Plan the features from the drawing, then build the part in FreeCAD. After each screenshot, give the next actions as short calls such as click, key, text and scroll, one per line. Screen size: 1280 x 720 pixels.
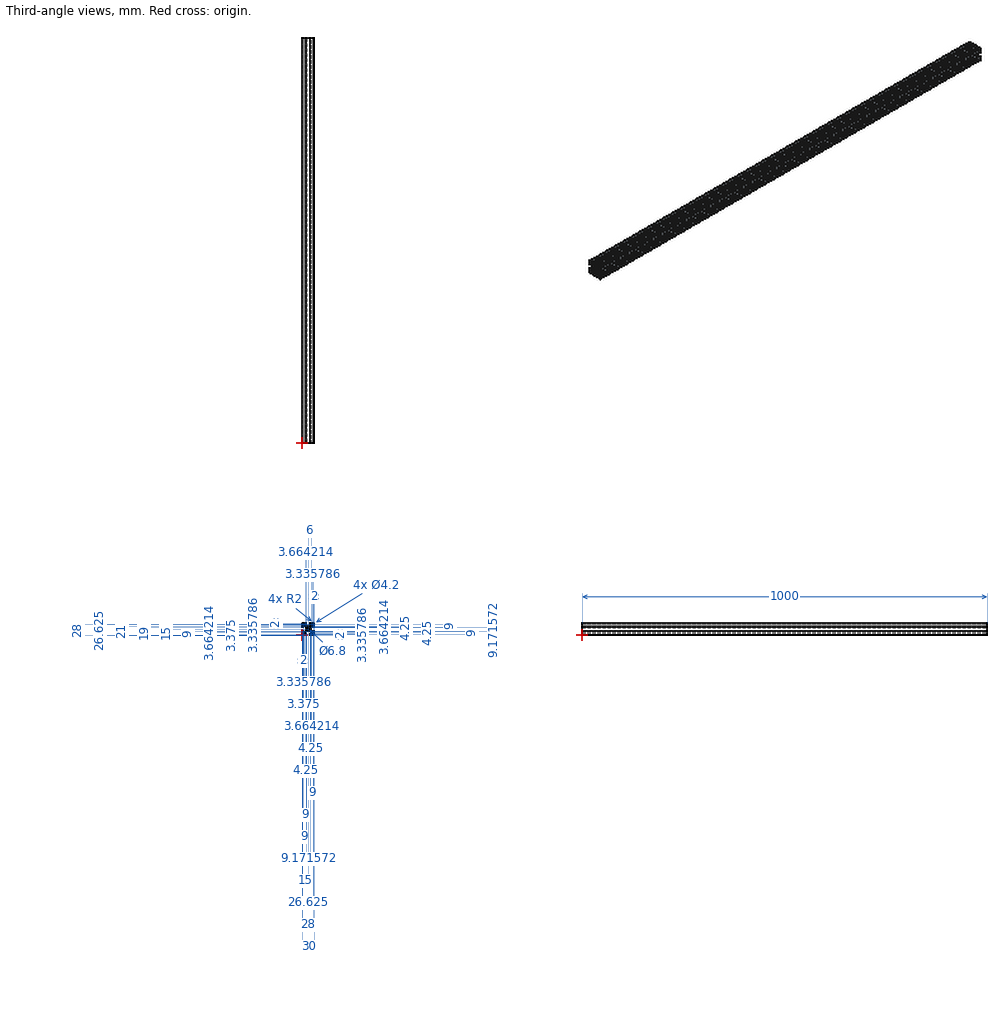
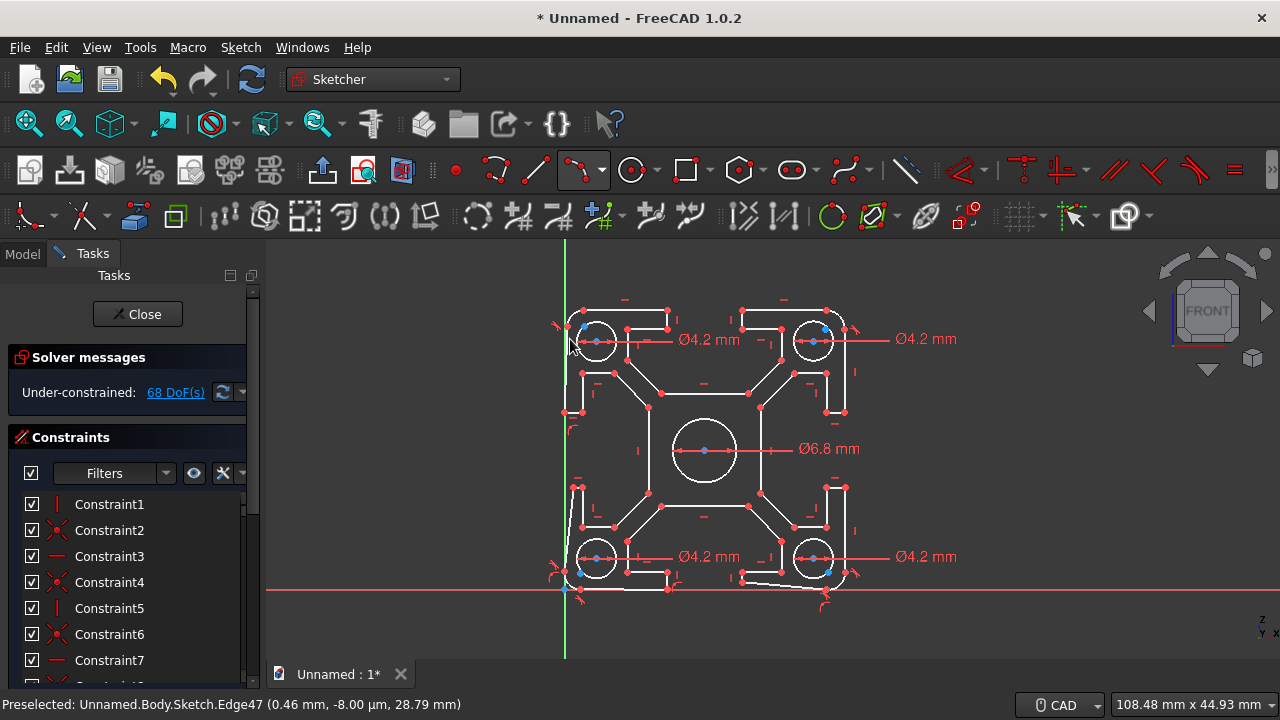
click(609, 310)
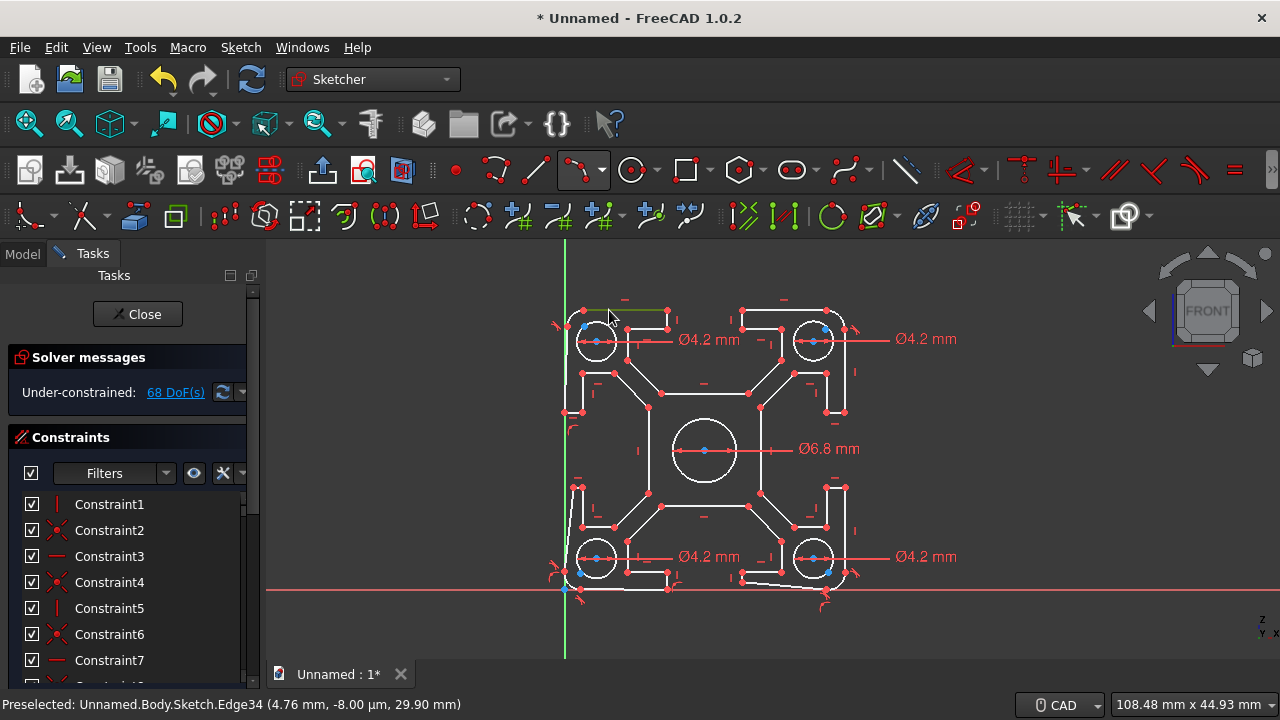
scroll(572, 315, up, 3)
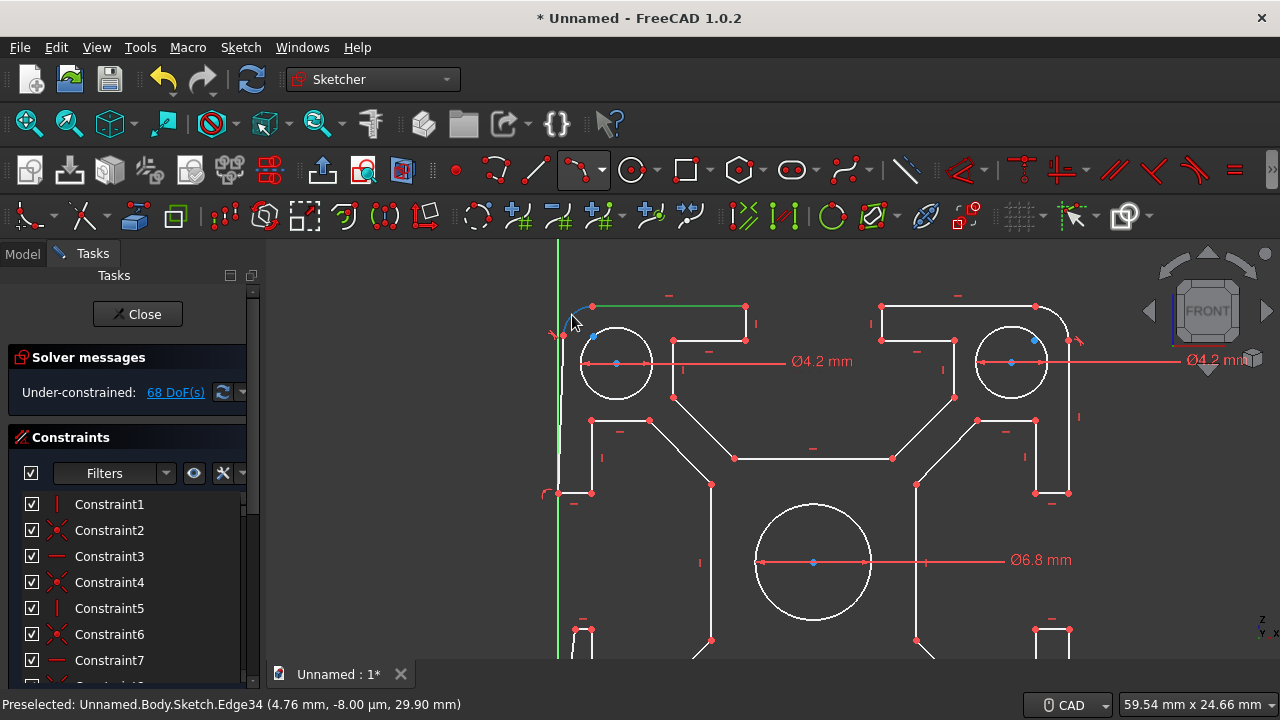
click(572, 315)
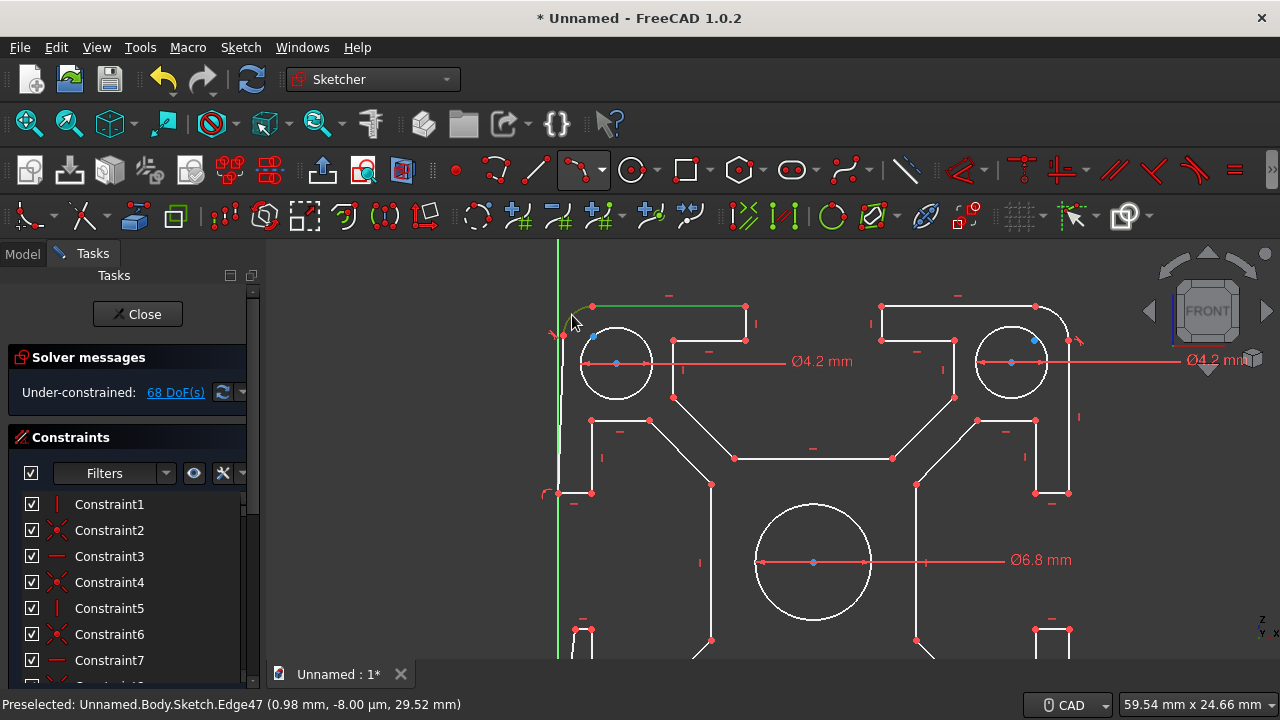
click(1196, 170)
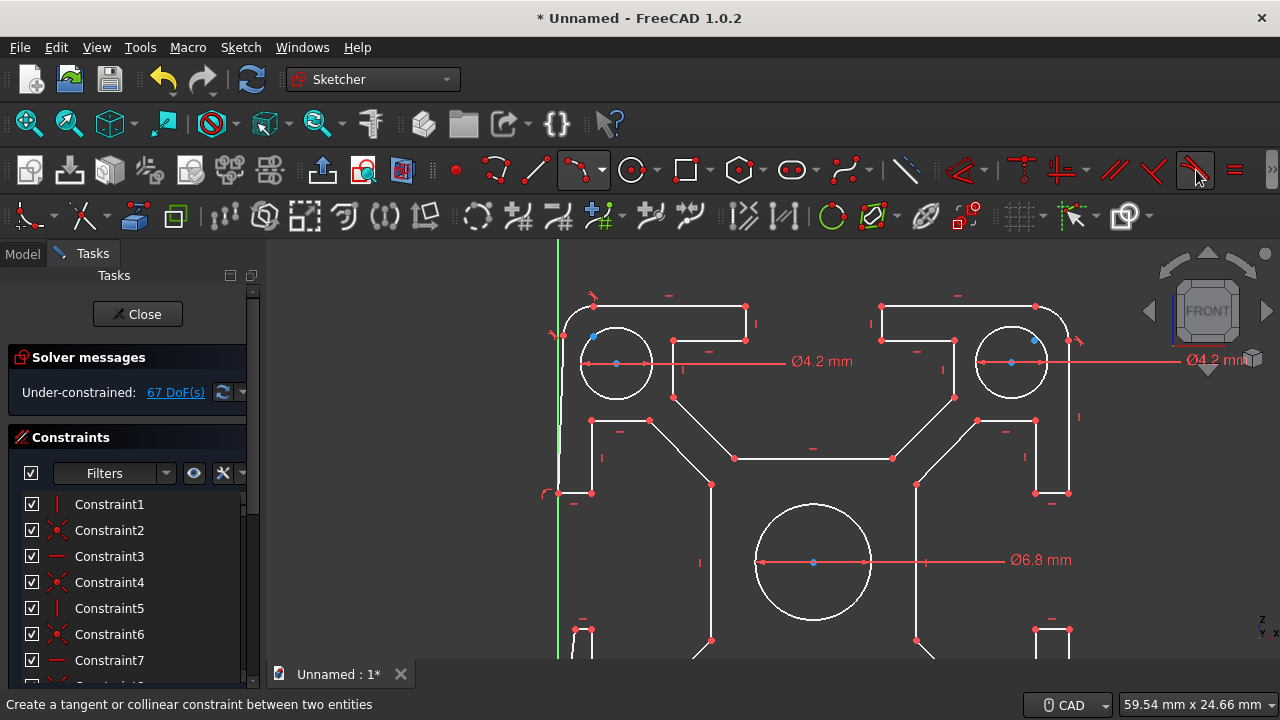
click(928, 306)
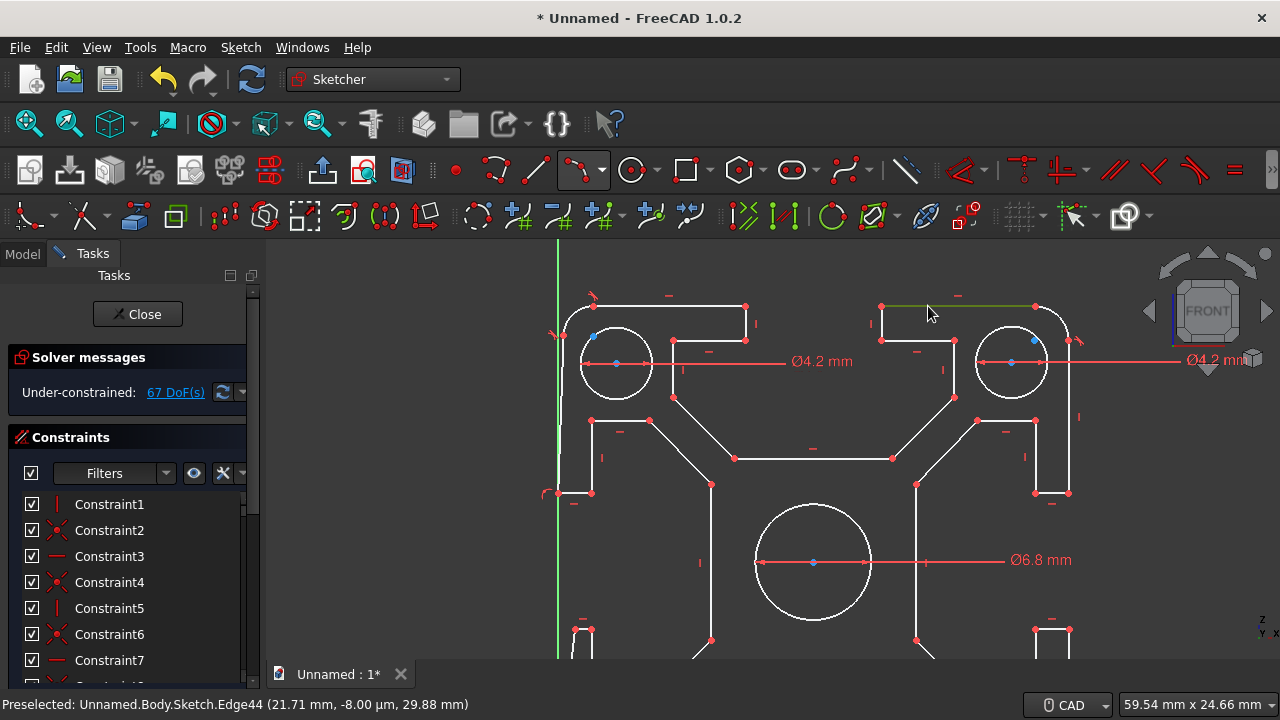
click(1065, 325)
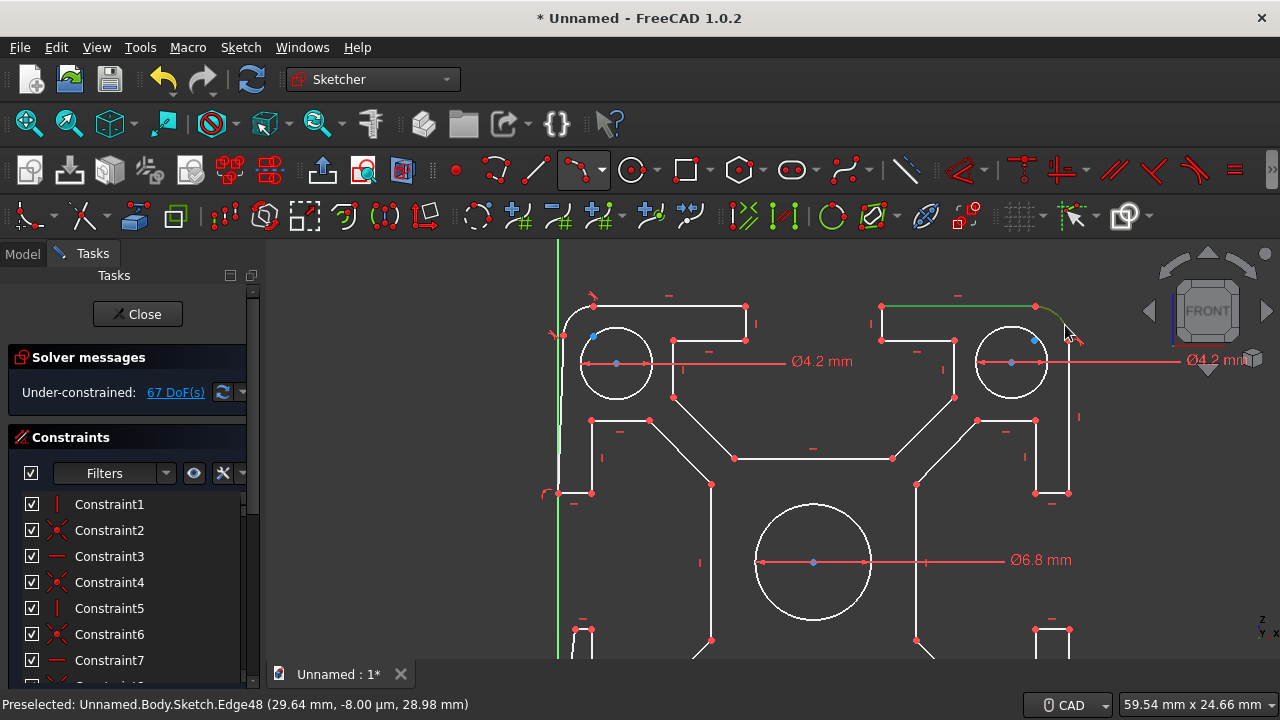
click(1196, 170)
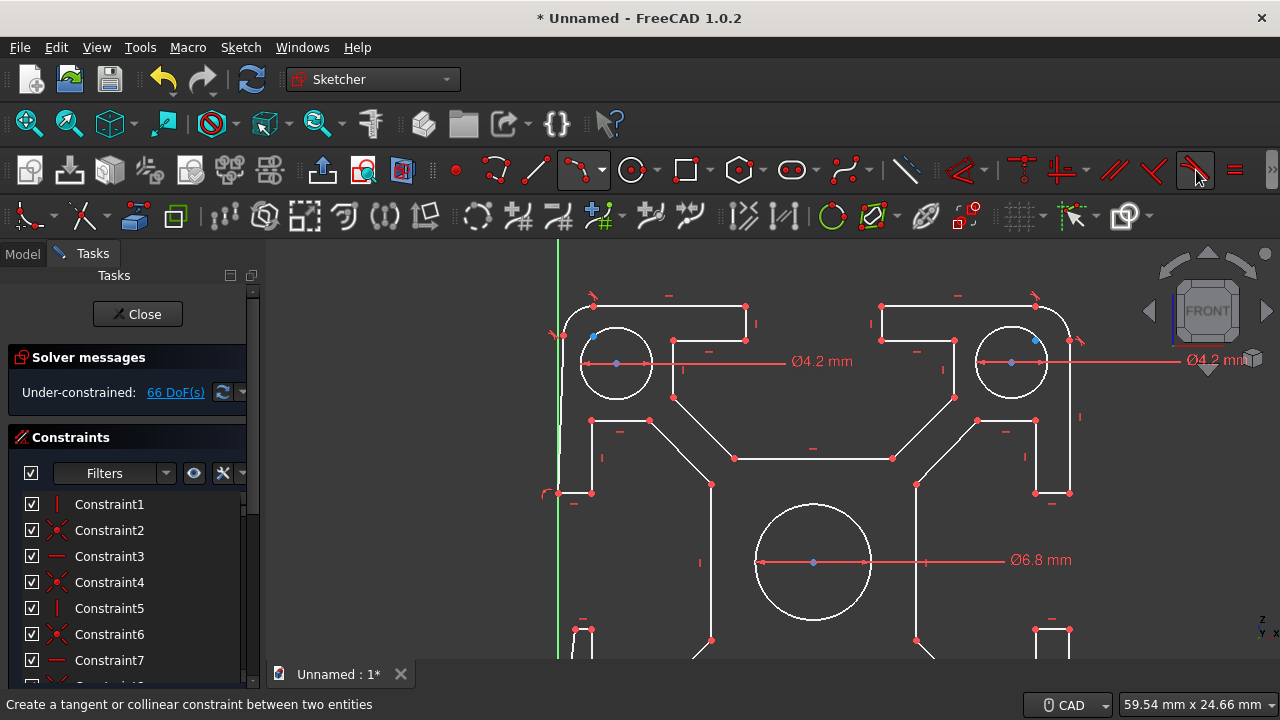
scroll(572, 314, down, 3)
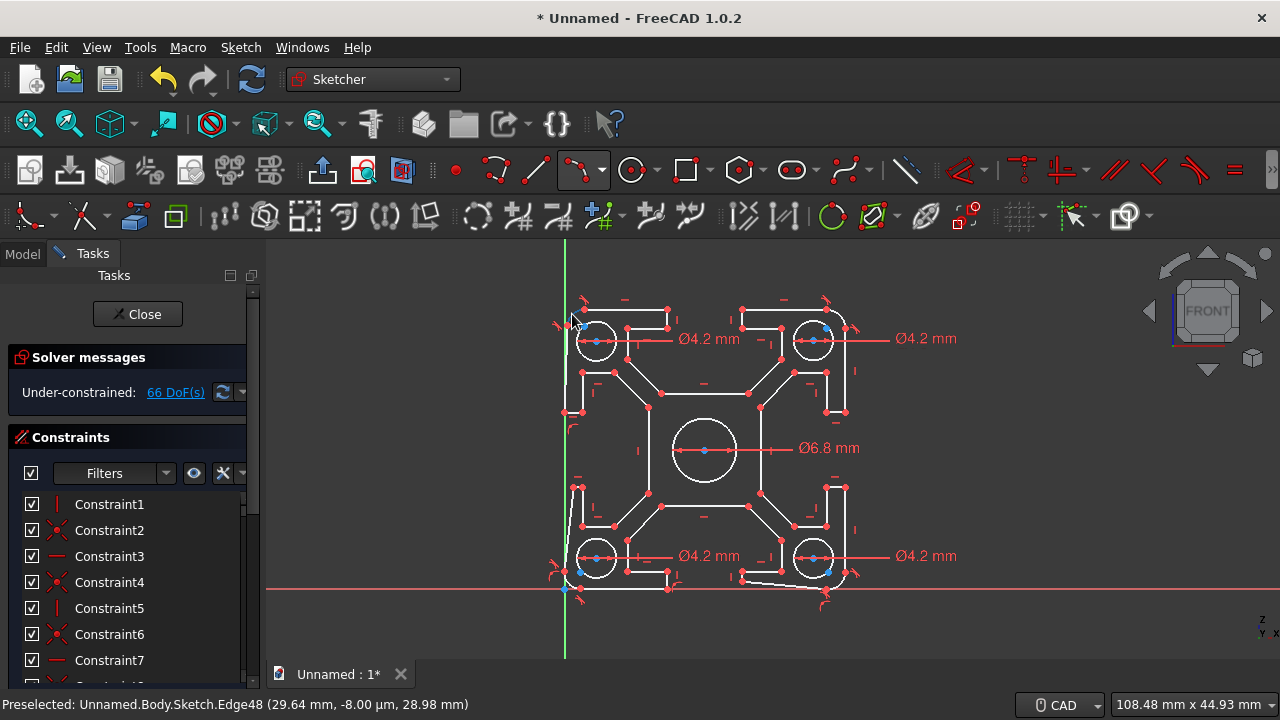
scroll(767, 584, up, 5)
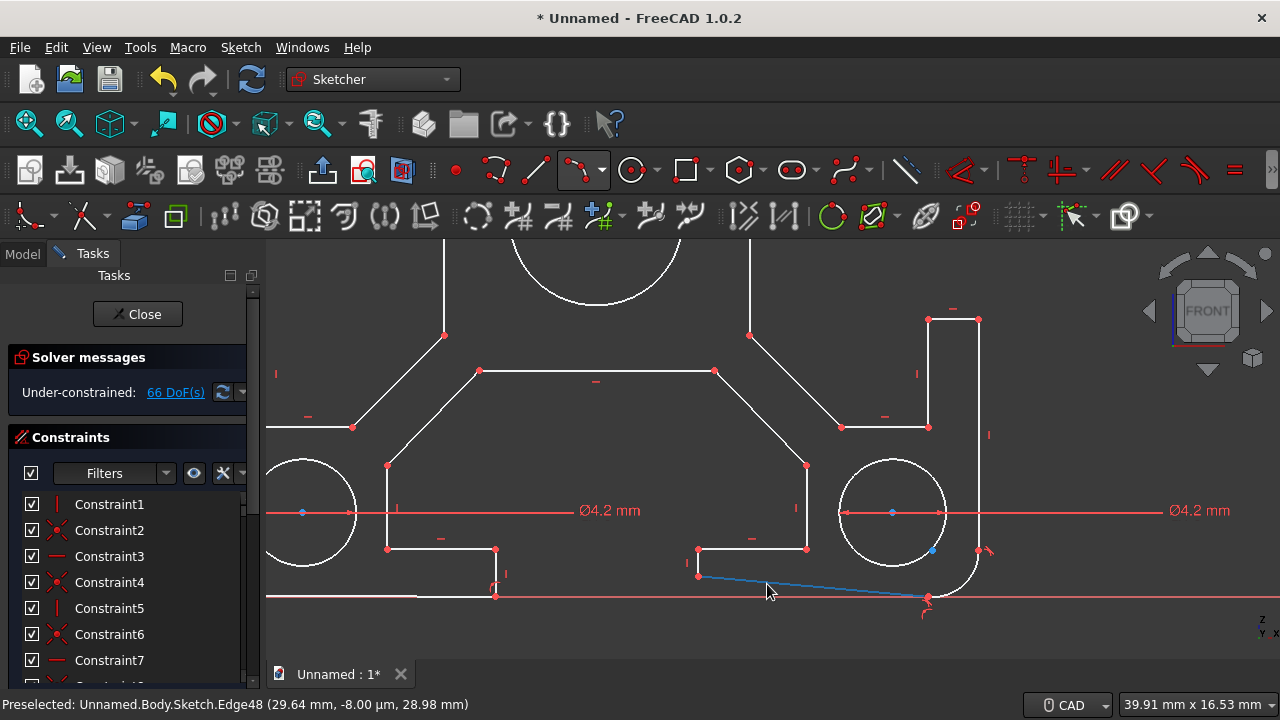
click(767, 582)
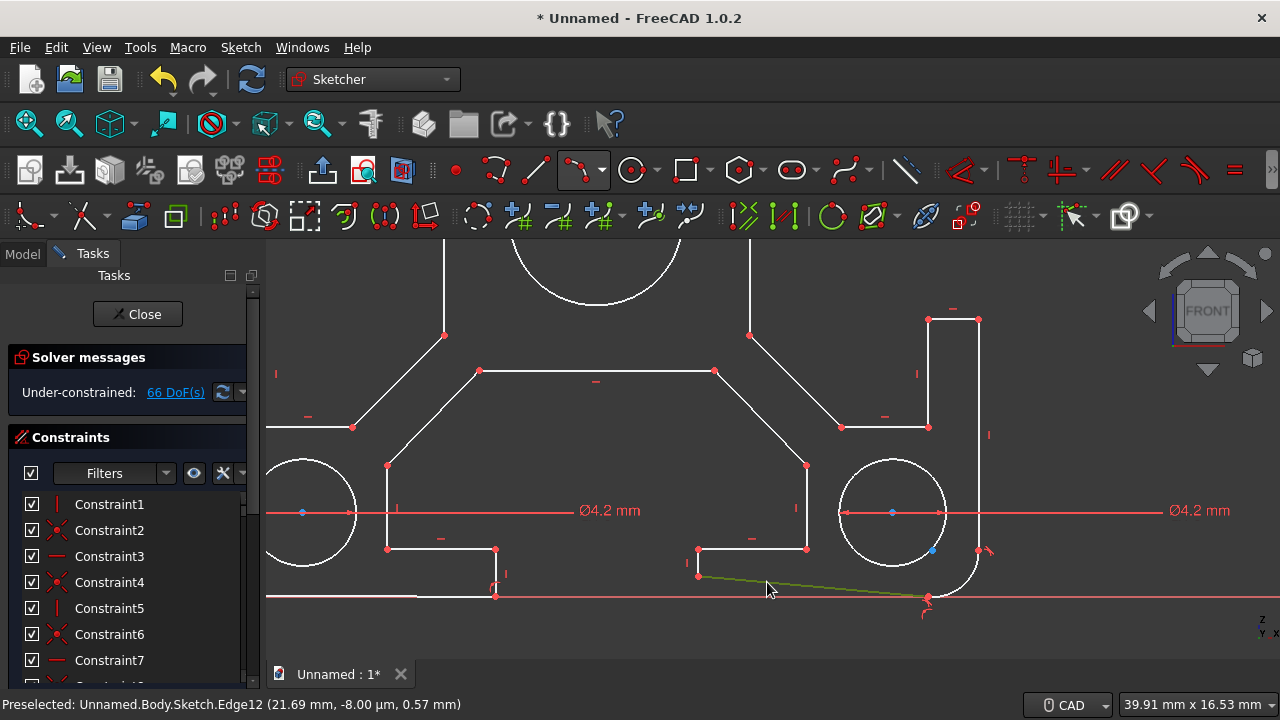
key(h)